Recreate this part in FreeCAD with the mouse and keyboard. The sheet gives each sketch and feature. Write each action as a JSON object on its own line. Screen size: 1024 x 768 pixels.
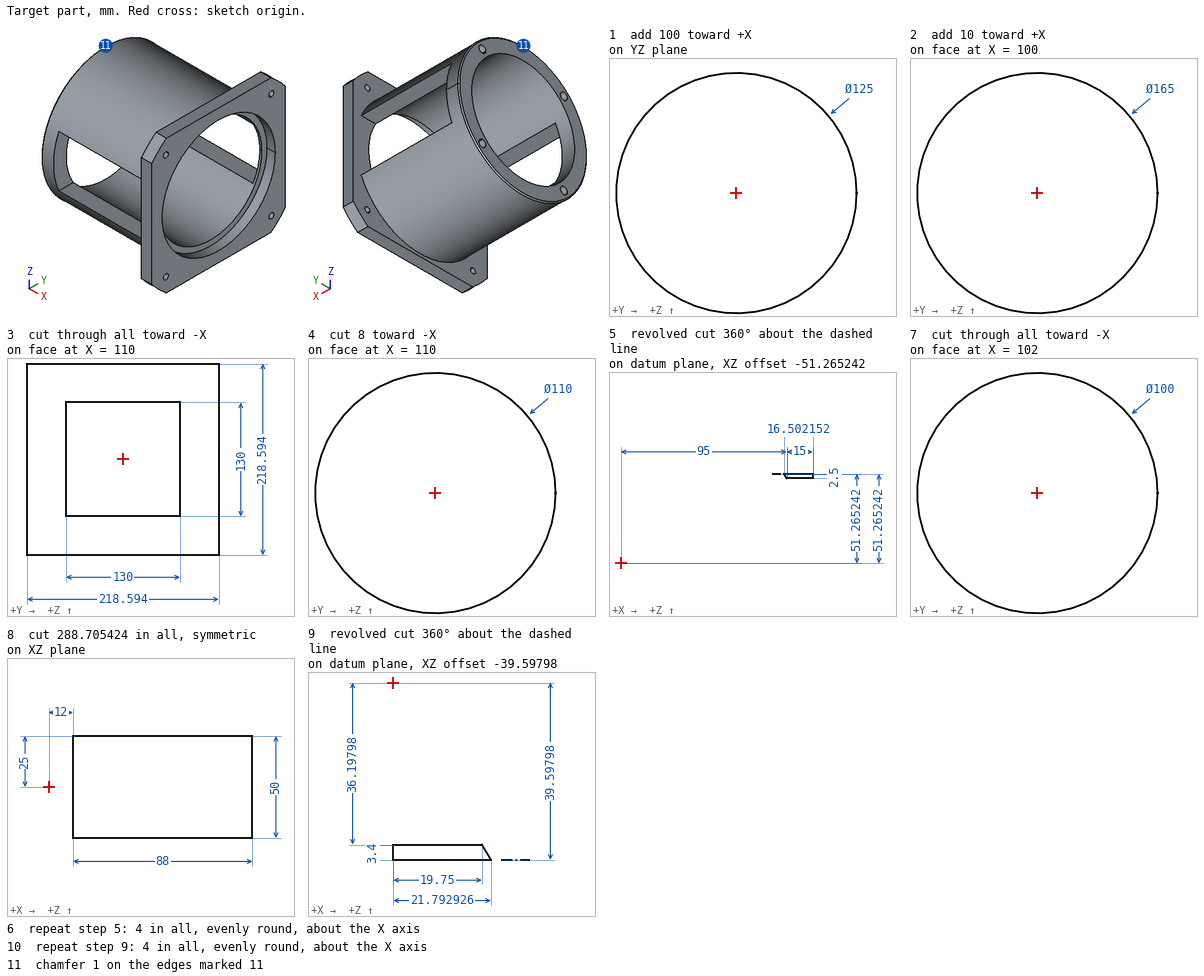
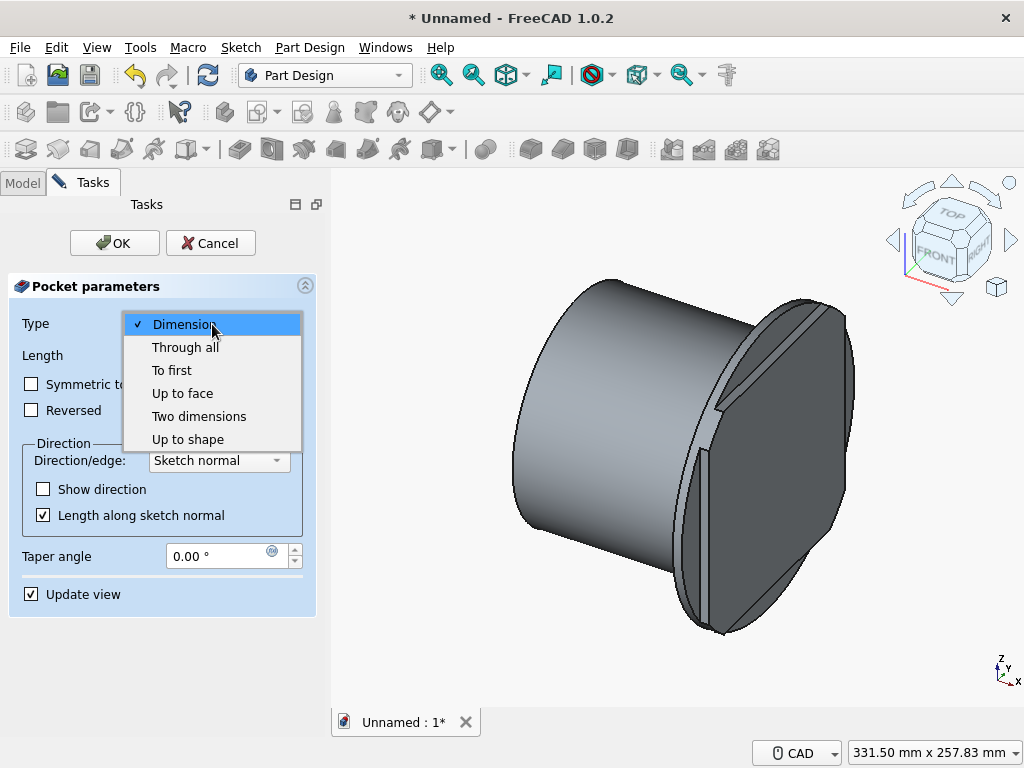
{"action": "left_click", "coordinate": [212, 348]}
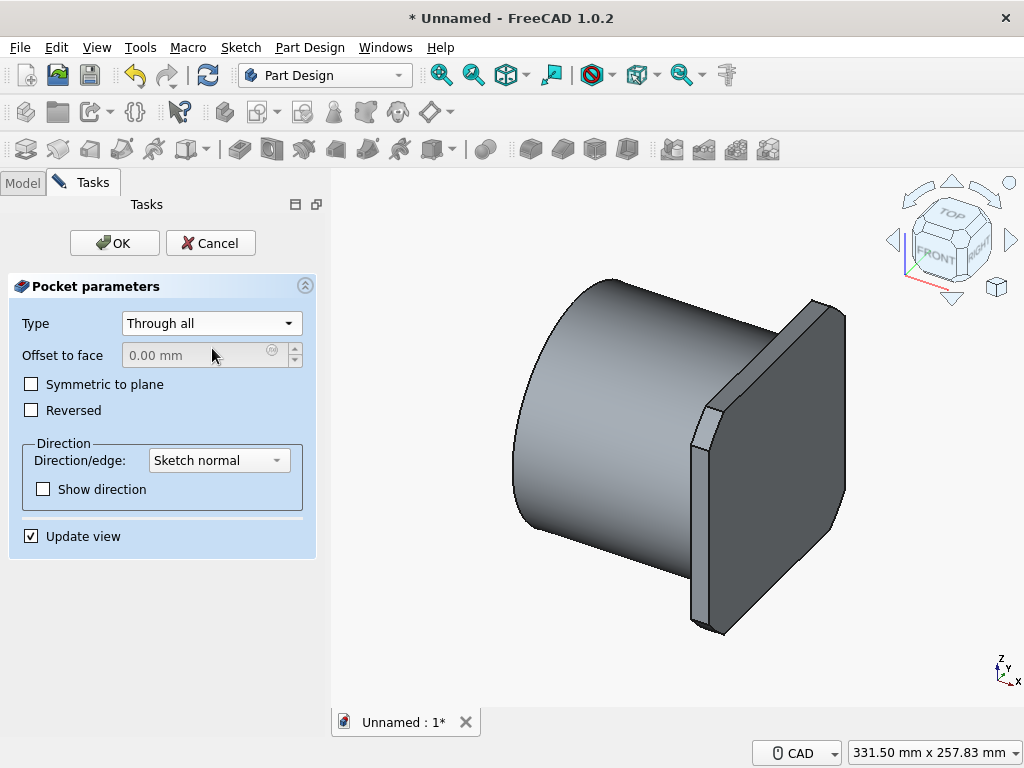
{"action": "left_click", "coordinate": [115, 243]}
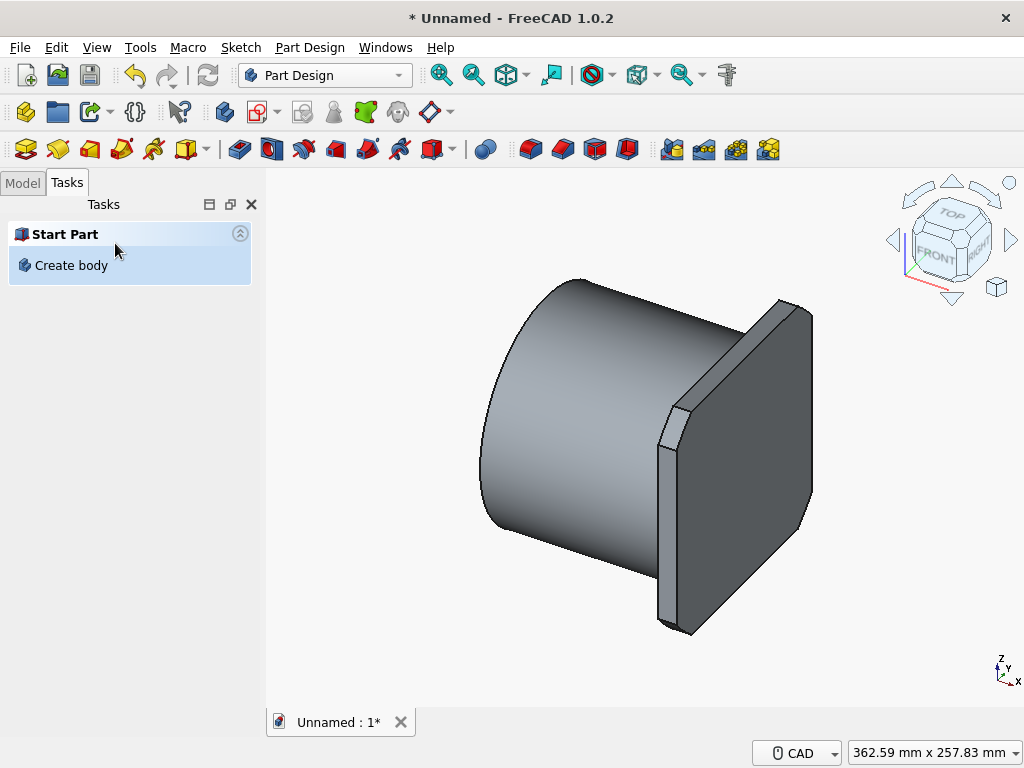
{"action": "left_click", "coordinate": [744, 470]}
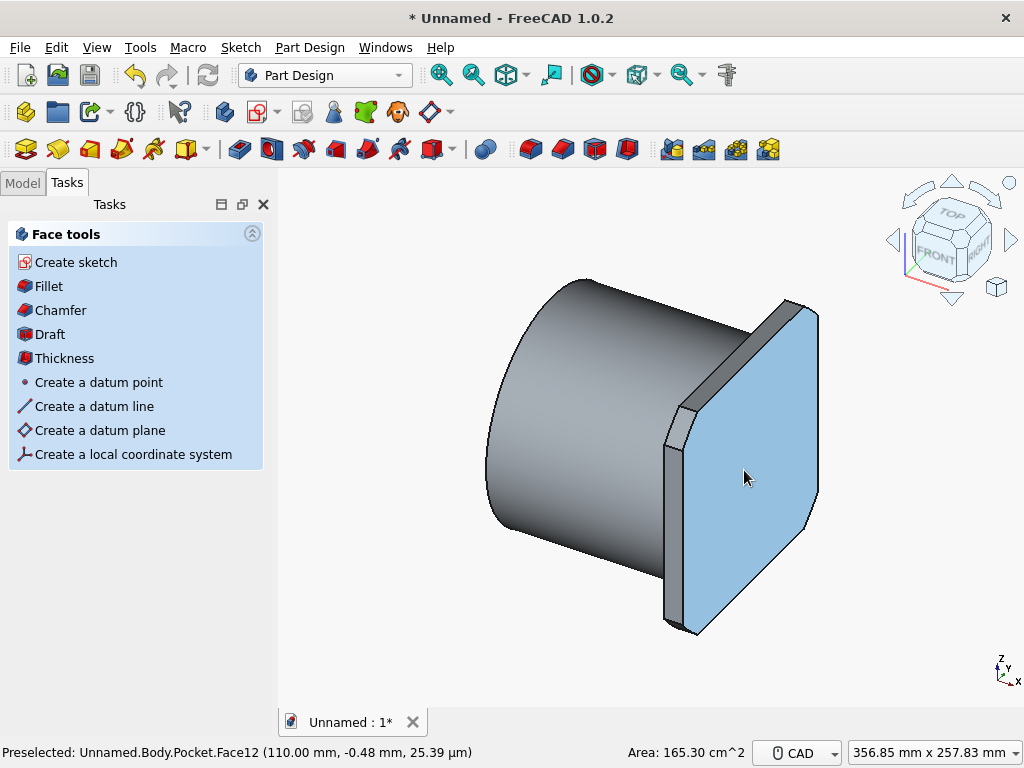
{"action": "left_click", "coordinate": [258, 112]}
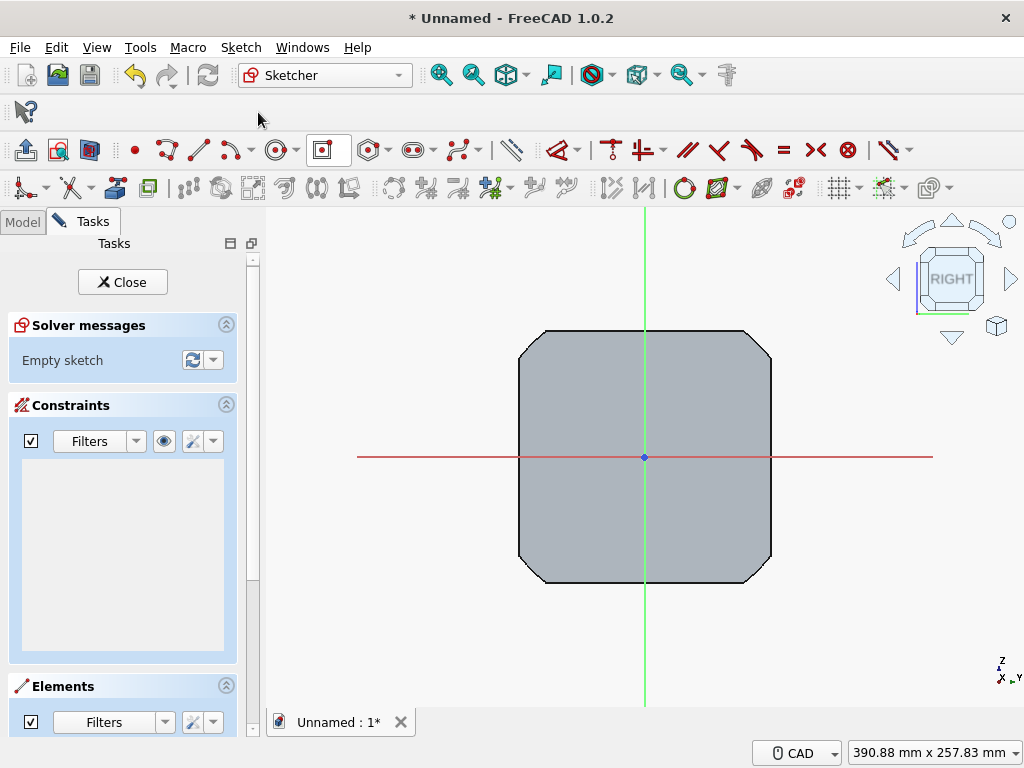
{"action": "scroll", "coordinate": [784, 457], "scroll_direction": "up", "scroll_amount": 2}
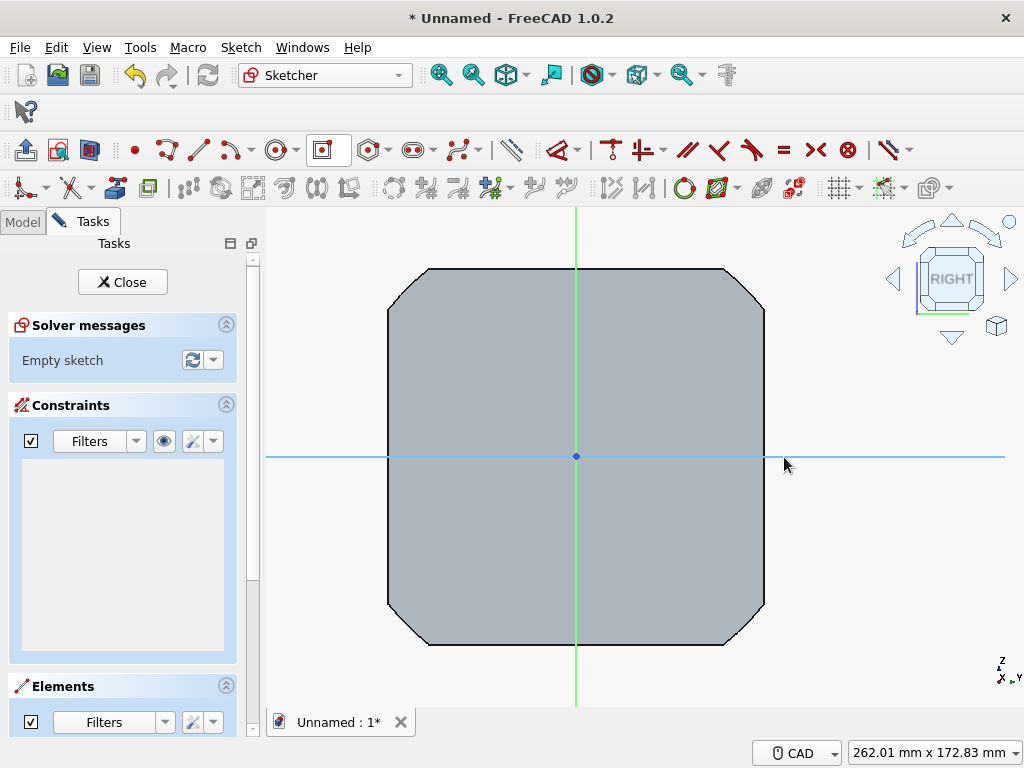
{"action": "left_click", "coordinate": [276, 150]}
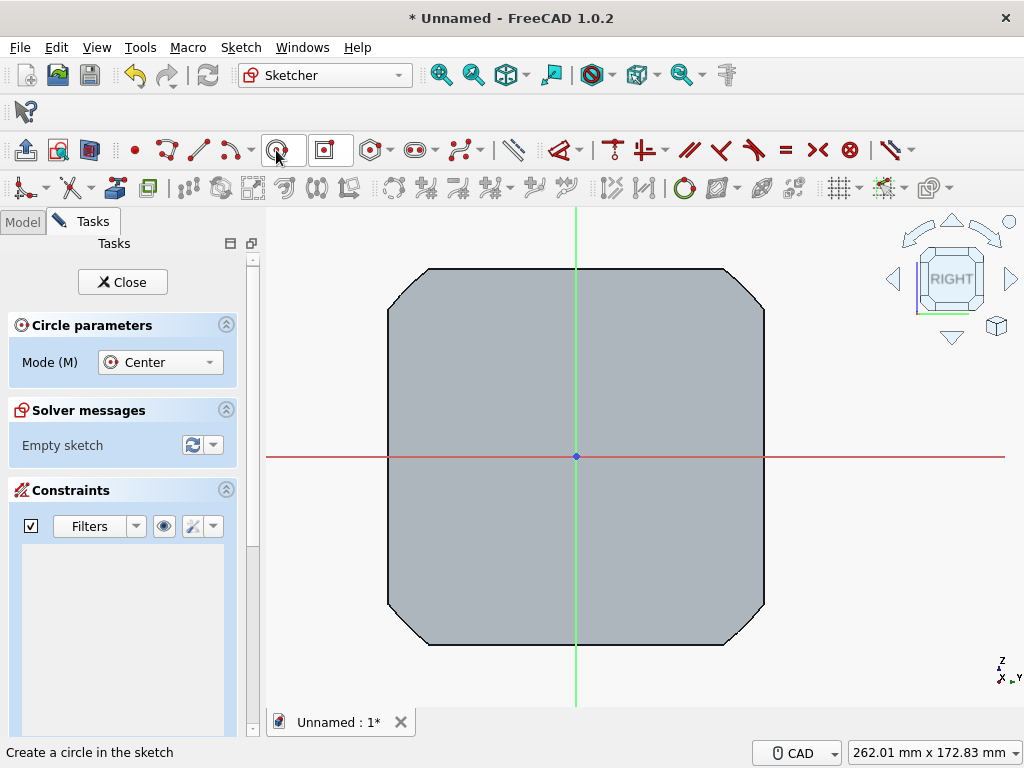
{"action": "left_click", "coordinate": [576, 457]}
{"action": "mouse_move", "coordinate": [689, 344]}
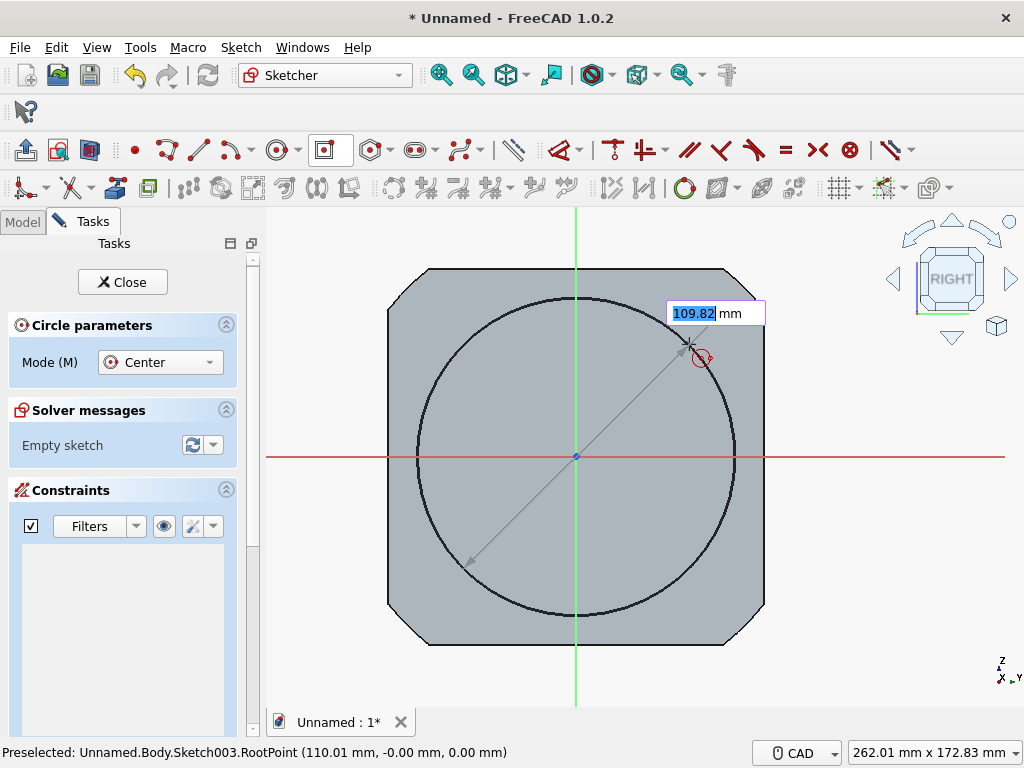
{"action": "type", "text": "110"}
{"action": "key", "text": "Return"}
{"action": "key", "text": "Escape"}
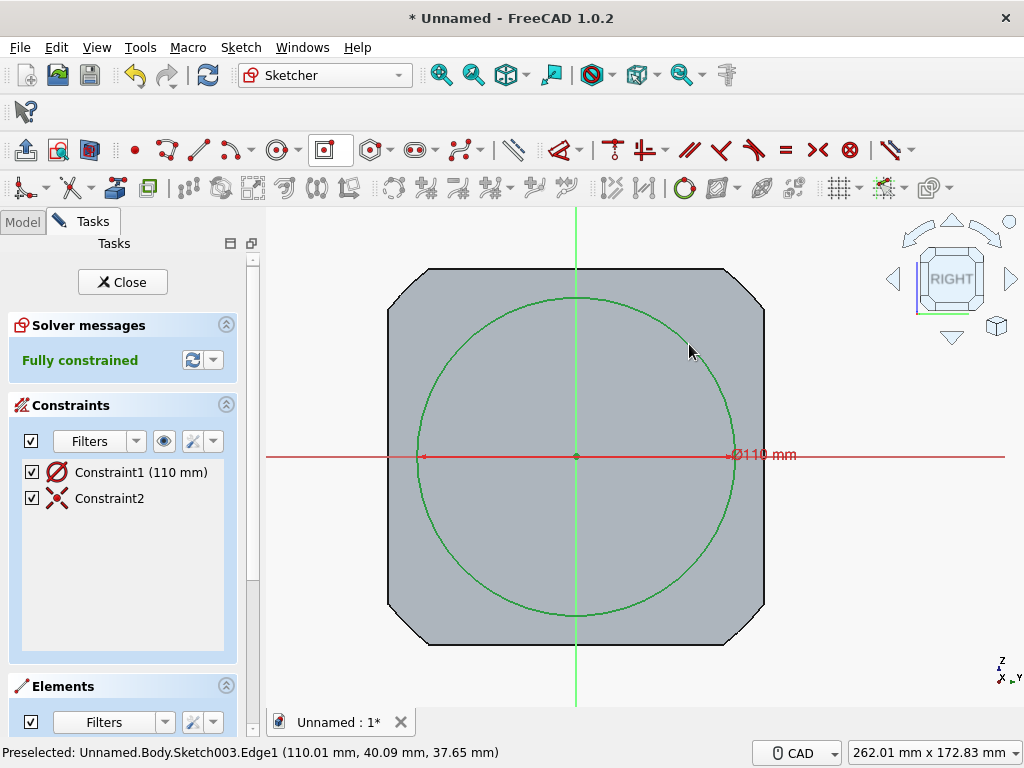
{"action": "left_click", "coordinate": [123, 282]}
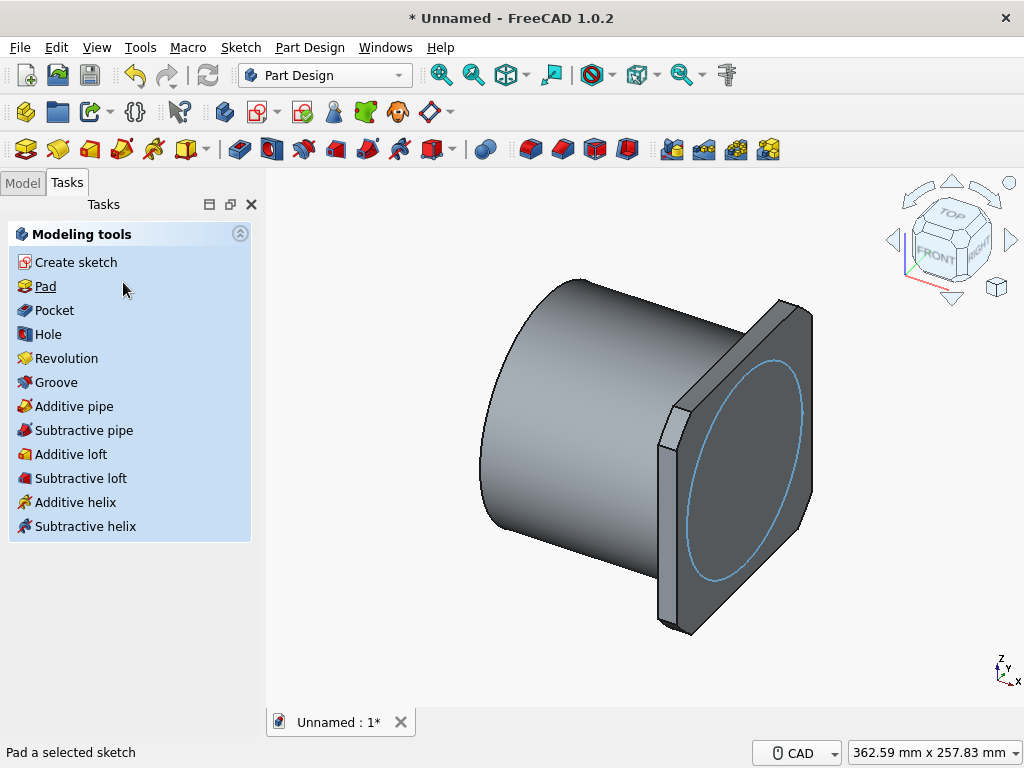
{"action": "left_click", "coordinate": [240, 150]}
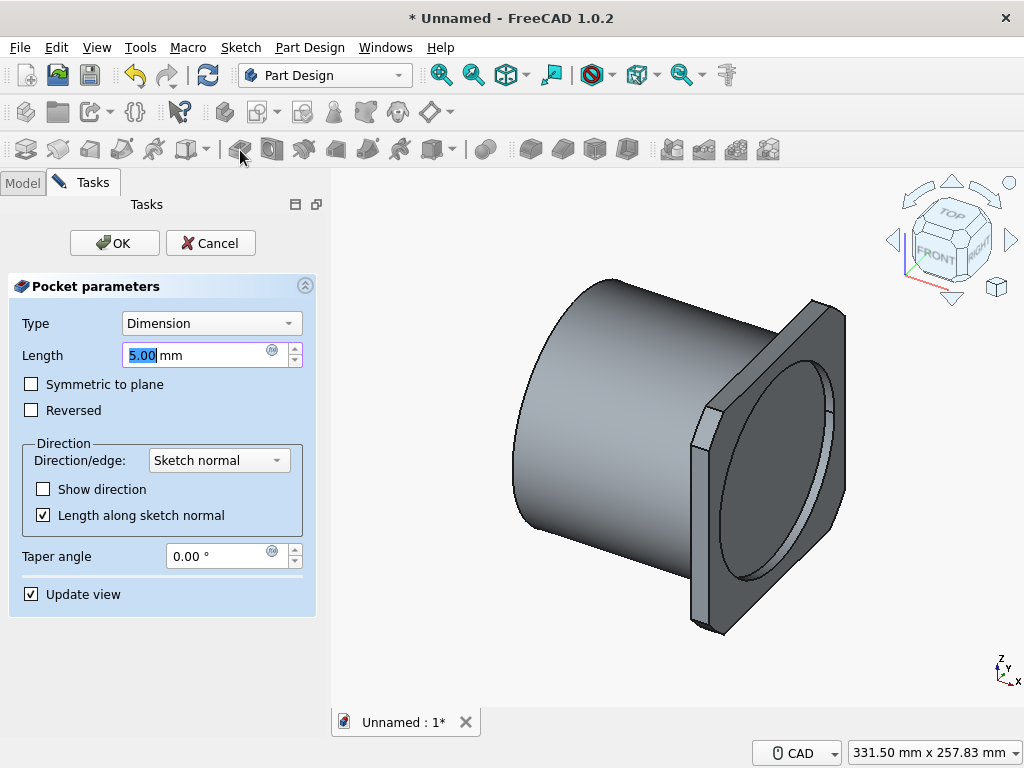
{"action": "type", "text": "8"}
{"action": "key", "text": "Tab"}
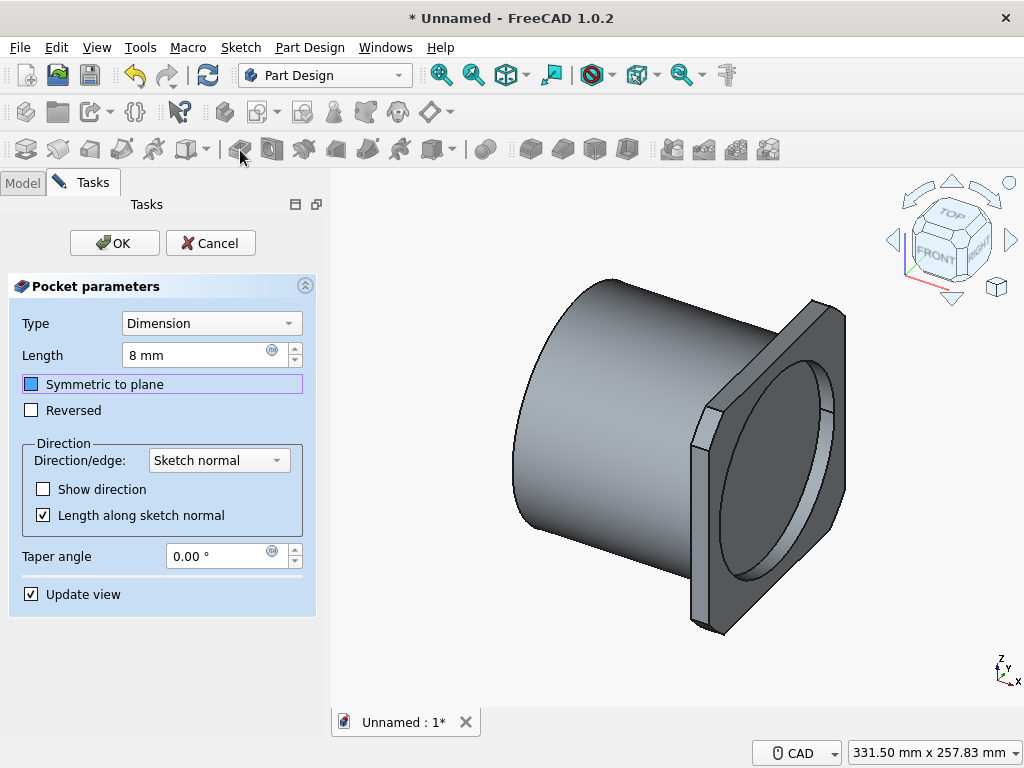
{"action": "left_click", "coordinate": [115, 243]}